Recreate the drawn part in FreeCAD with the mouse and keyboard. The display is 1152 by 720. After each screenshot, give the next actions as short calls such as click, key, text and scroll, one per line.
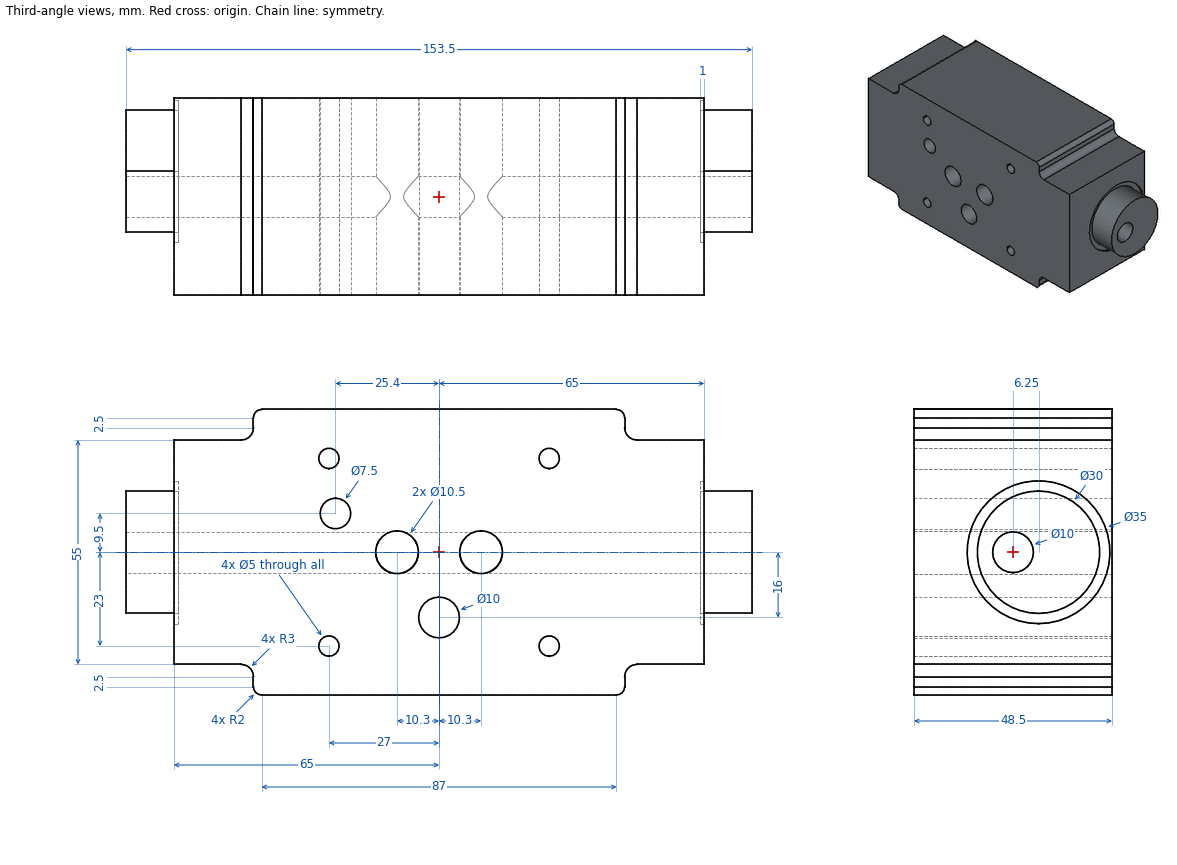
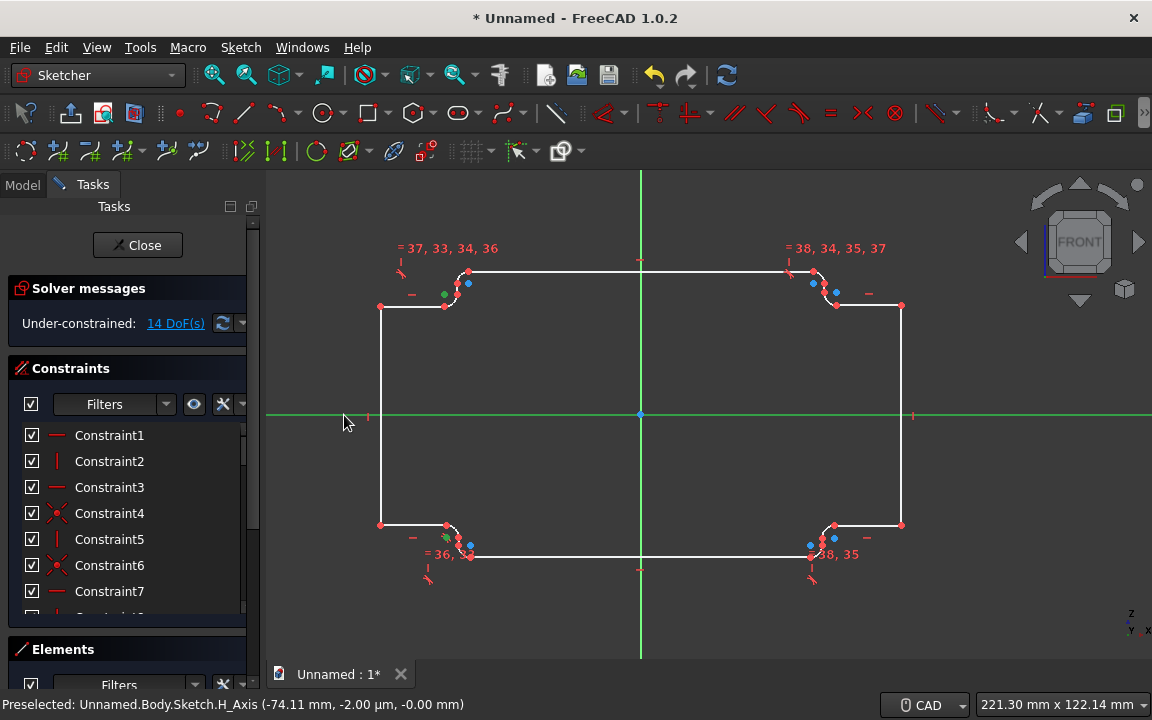
click(864, 114)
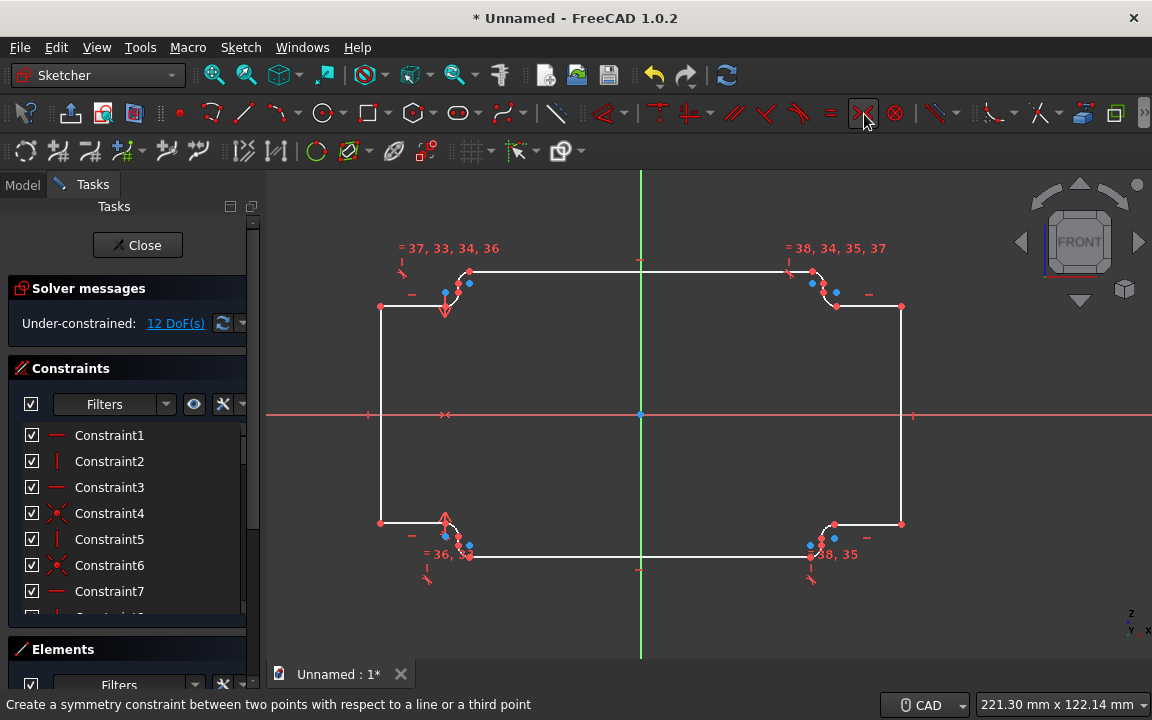
click(445, 293)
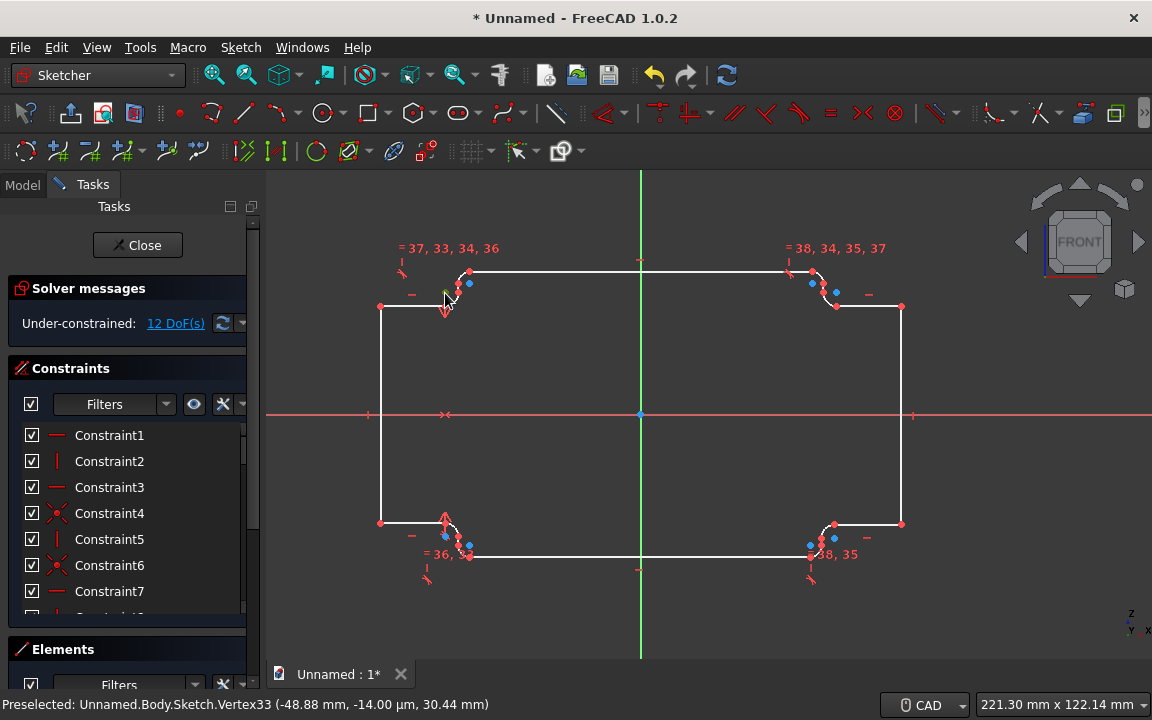
click(837, 293)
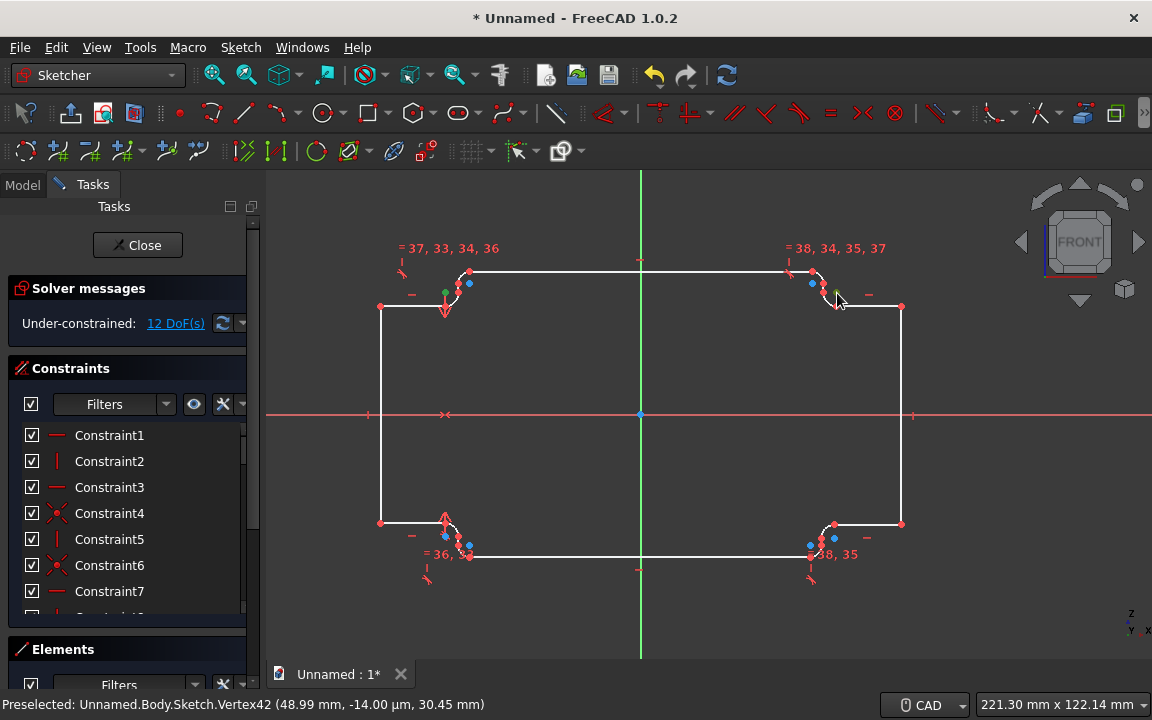
click(641, 600)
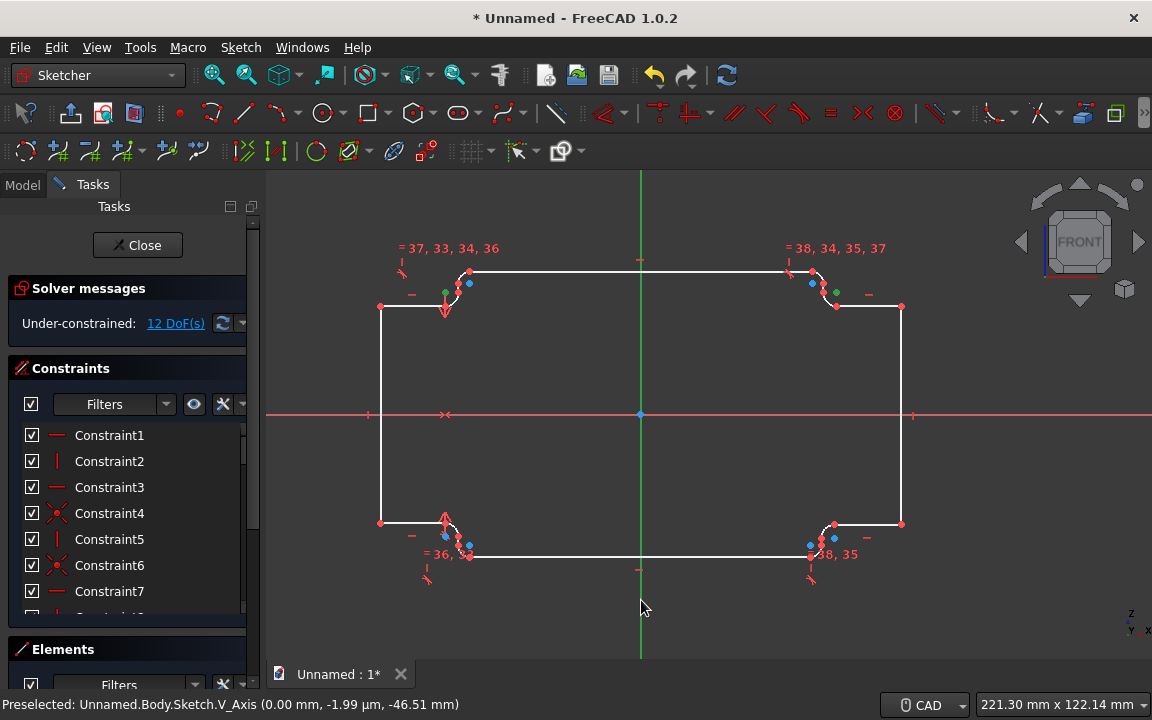
click(864, 114)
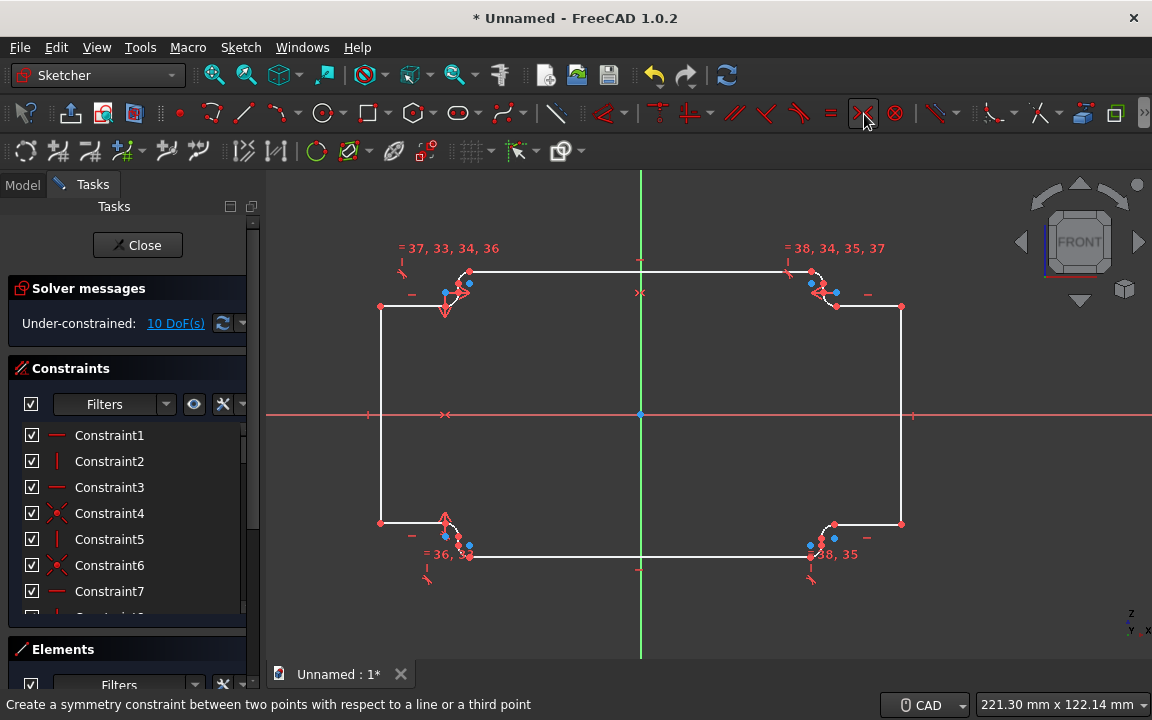
click(445, 537)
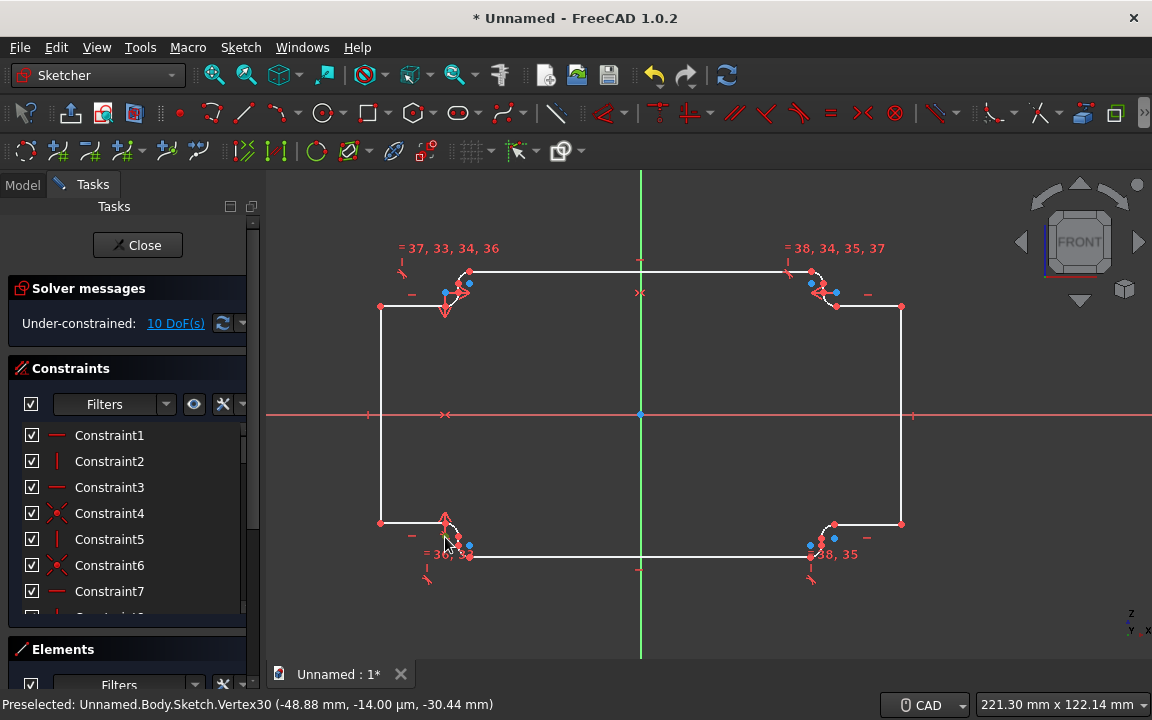
click(835, 538)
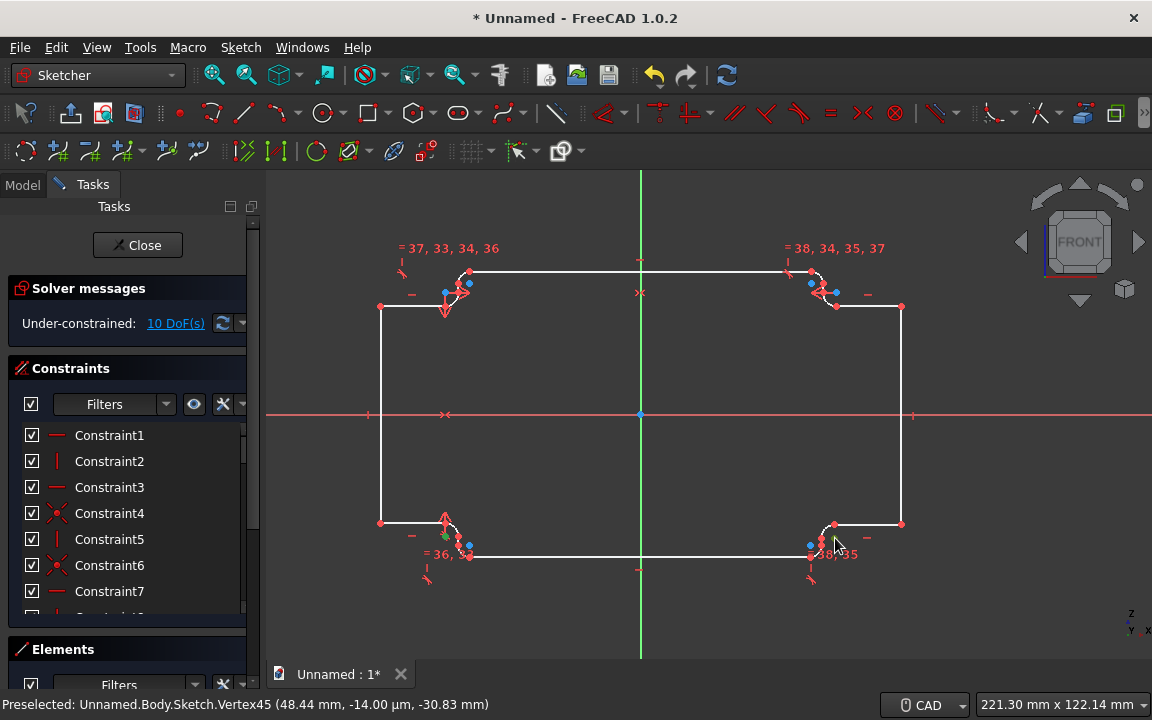
click(641, 600)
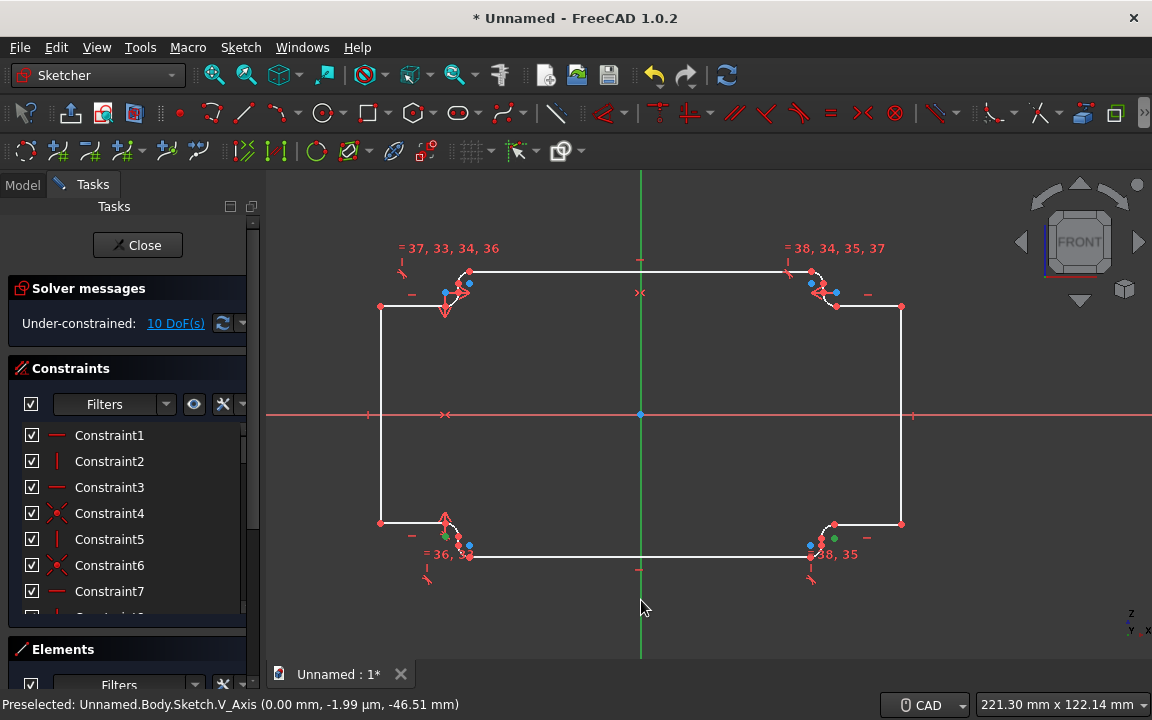
click(864, 114)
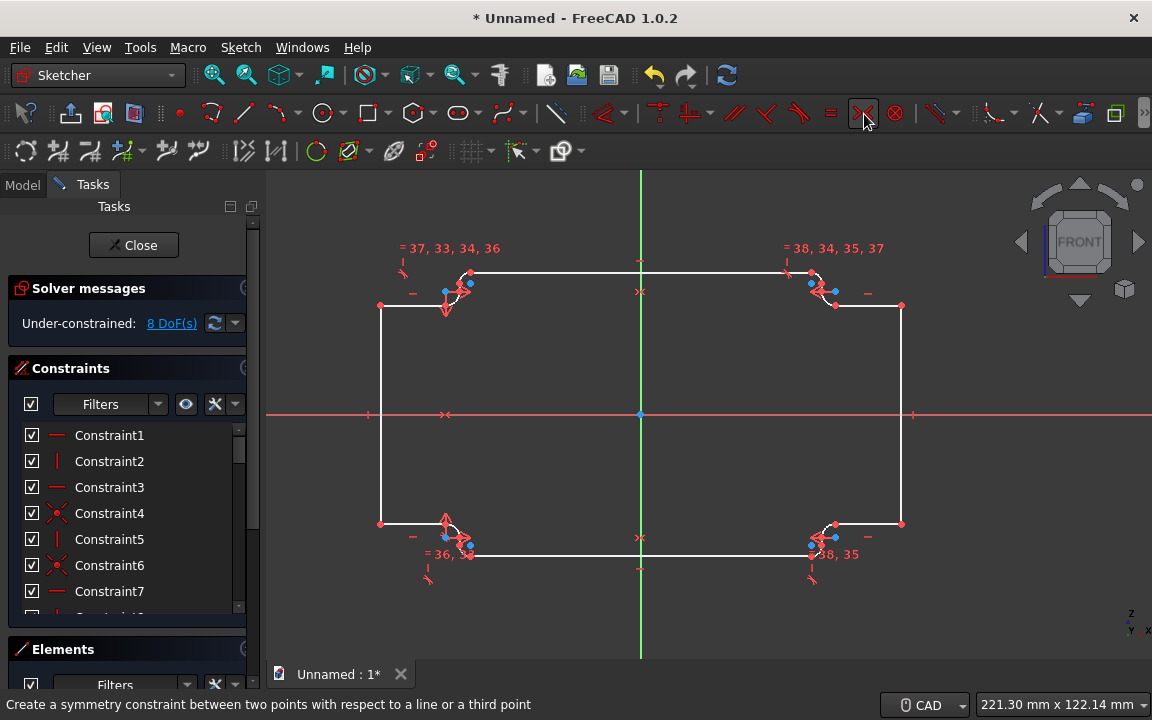
scroll(463, 553, up, 9)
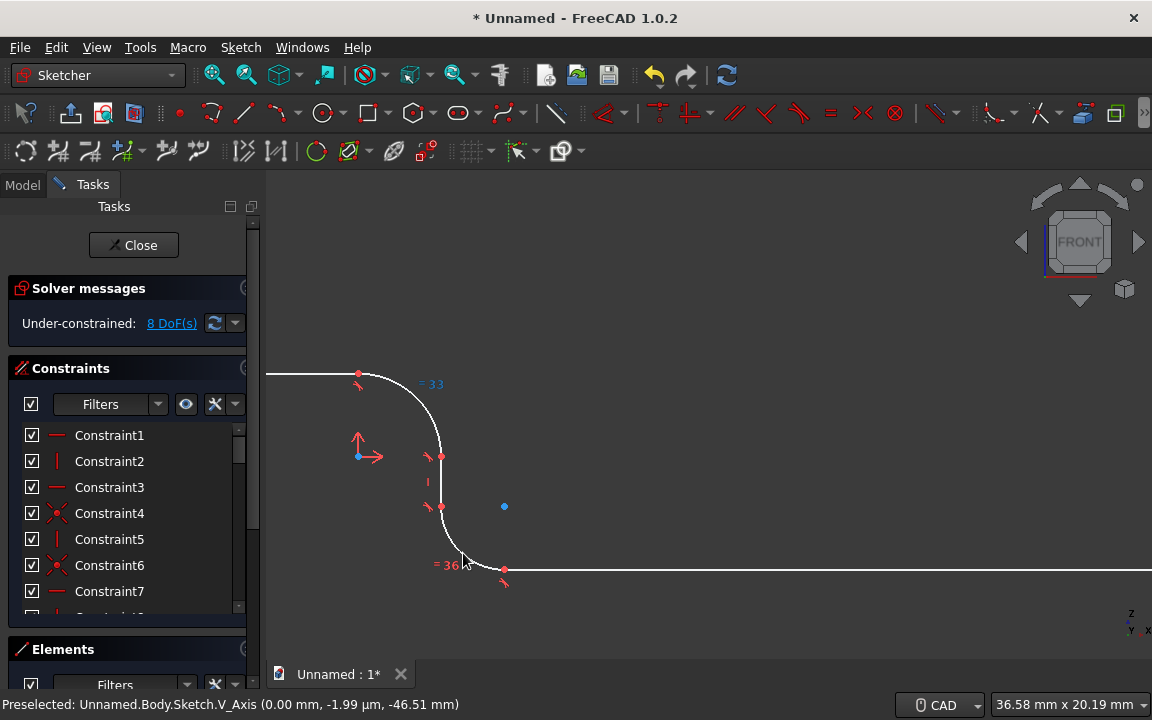
click(460, 551)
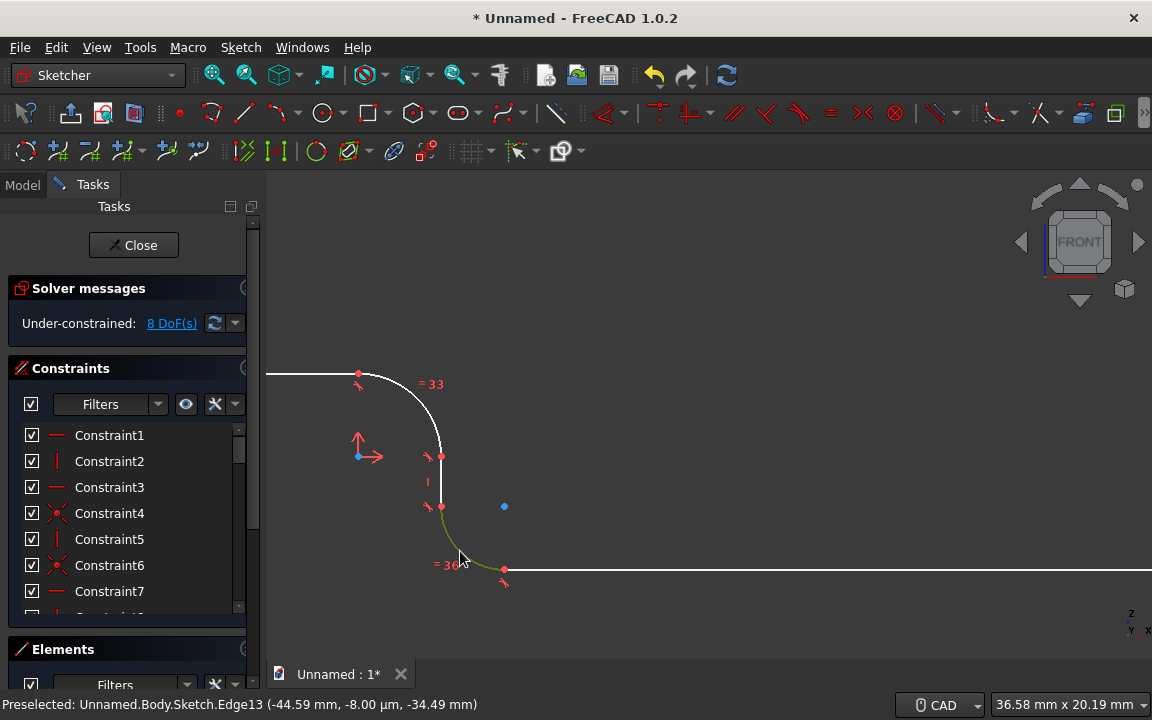
click(626, 114)